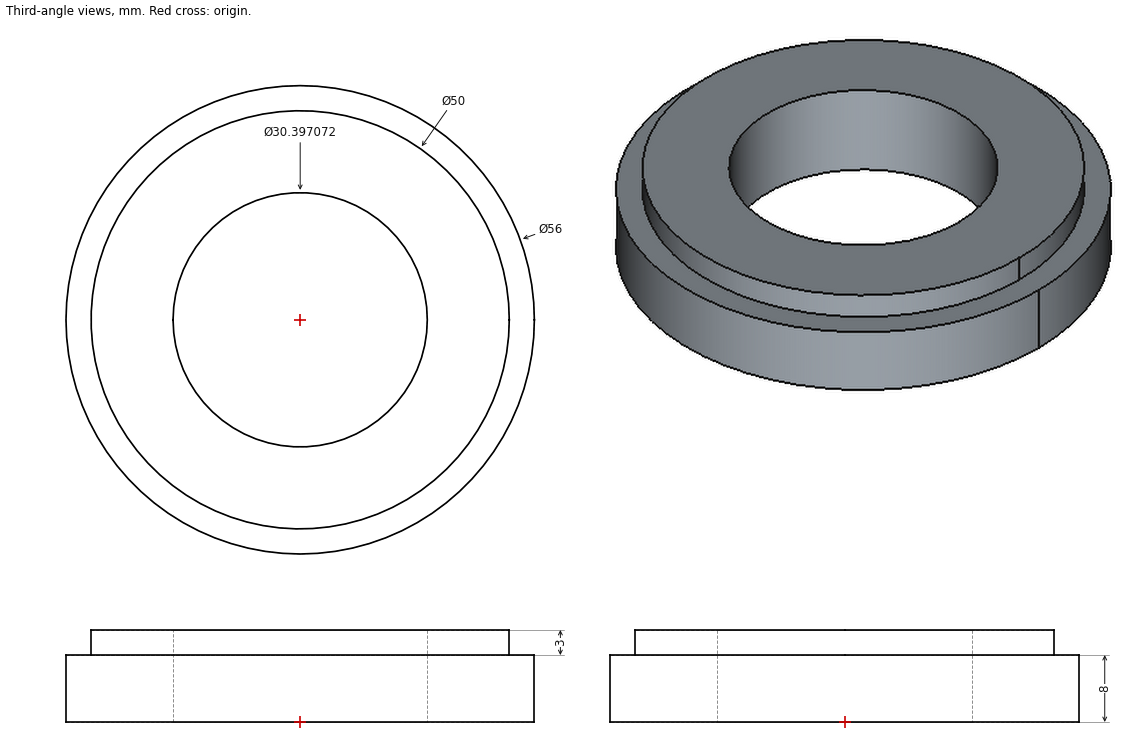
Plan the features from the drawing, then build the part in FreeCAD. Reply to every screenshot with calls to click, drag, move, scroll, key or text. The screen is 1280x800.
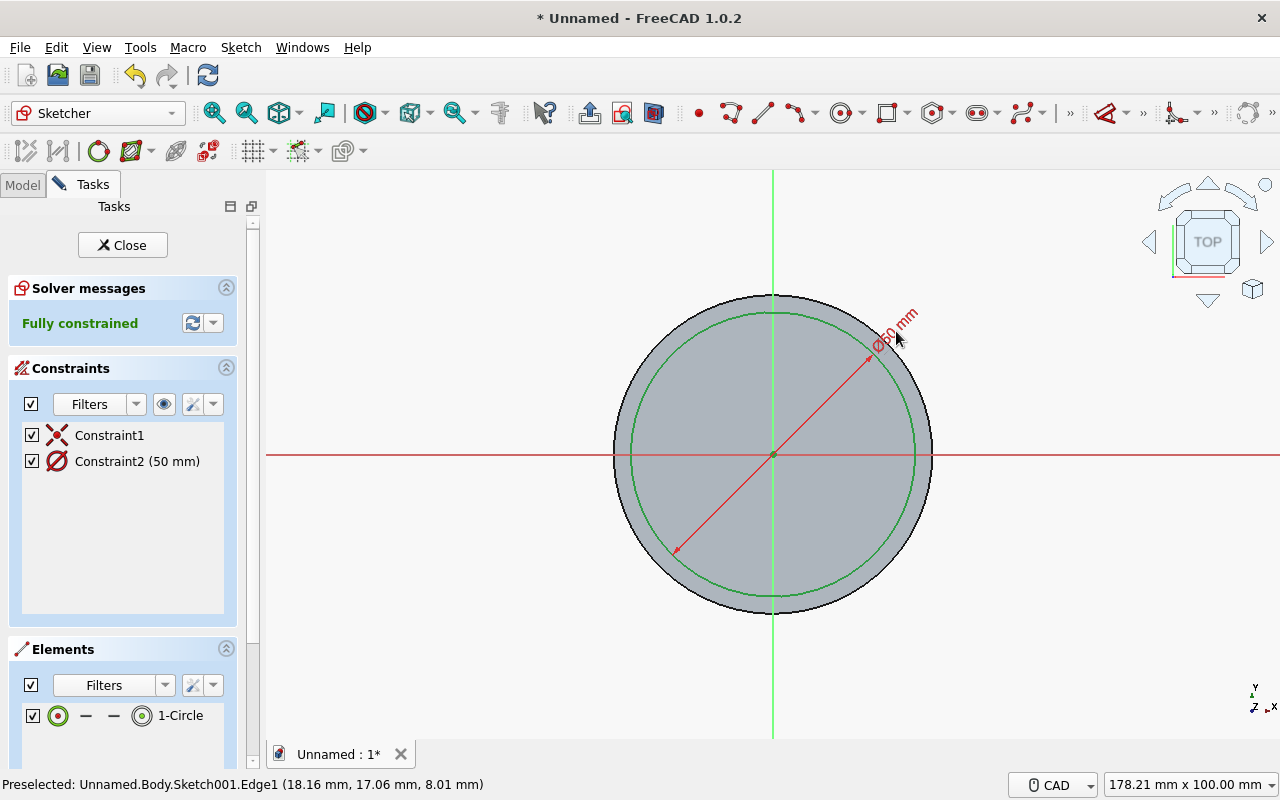
click(123, 245)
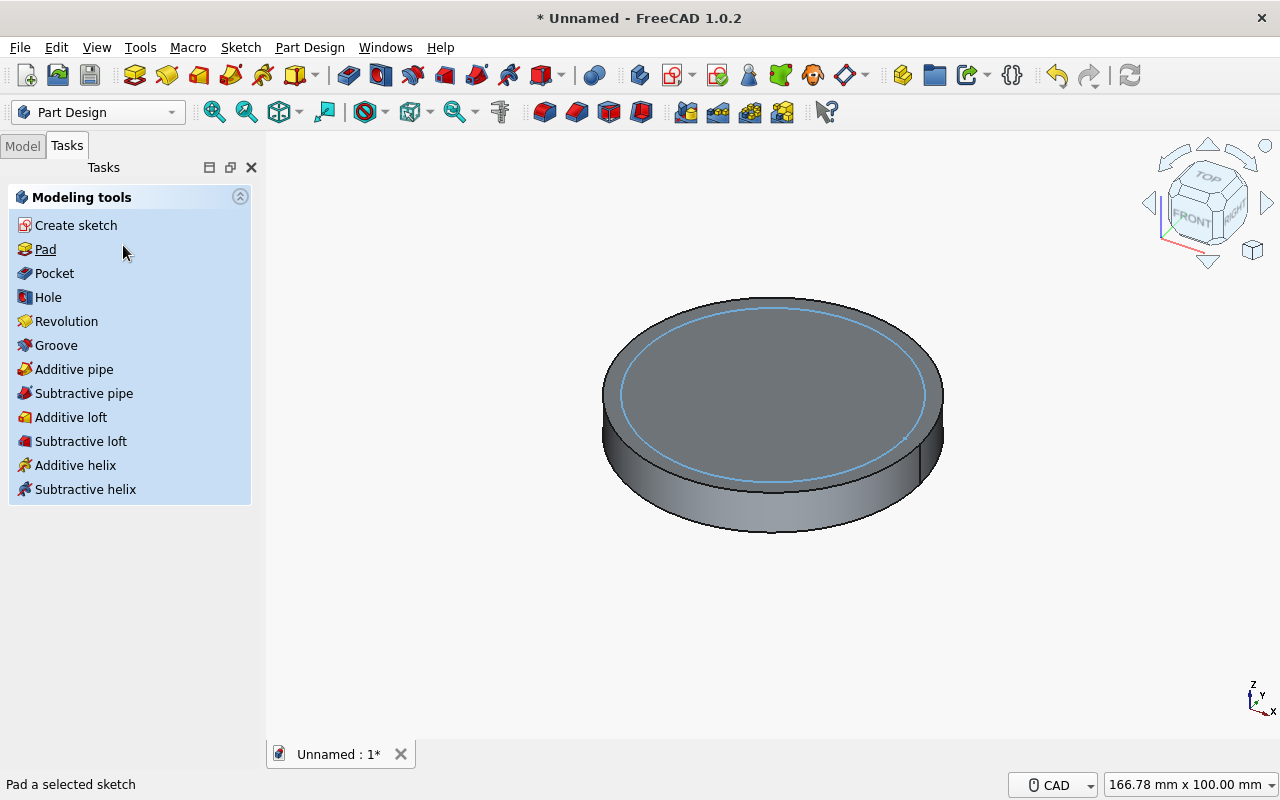
click(136, 76)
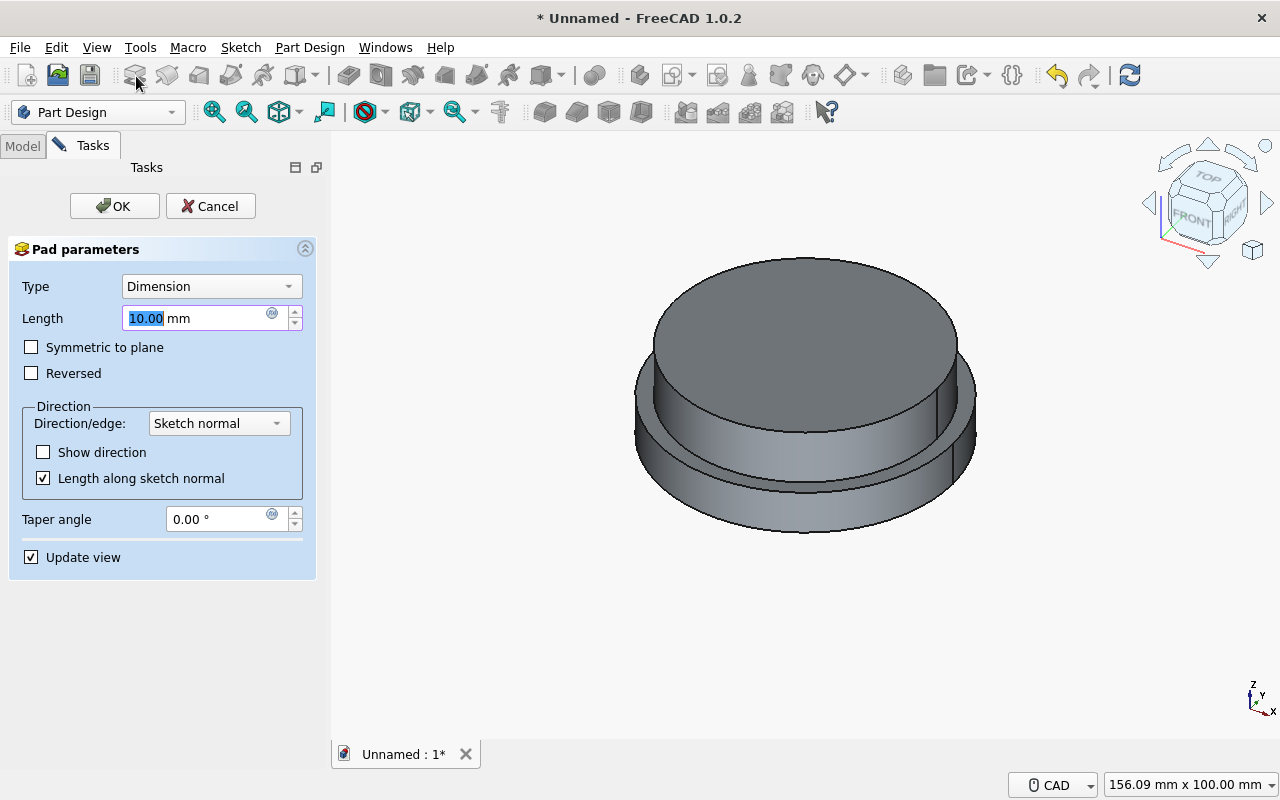
text(3)
key(Tab)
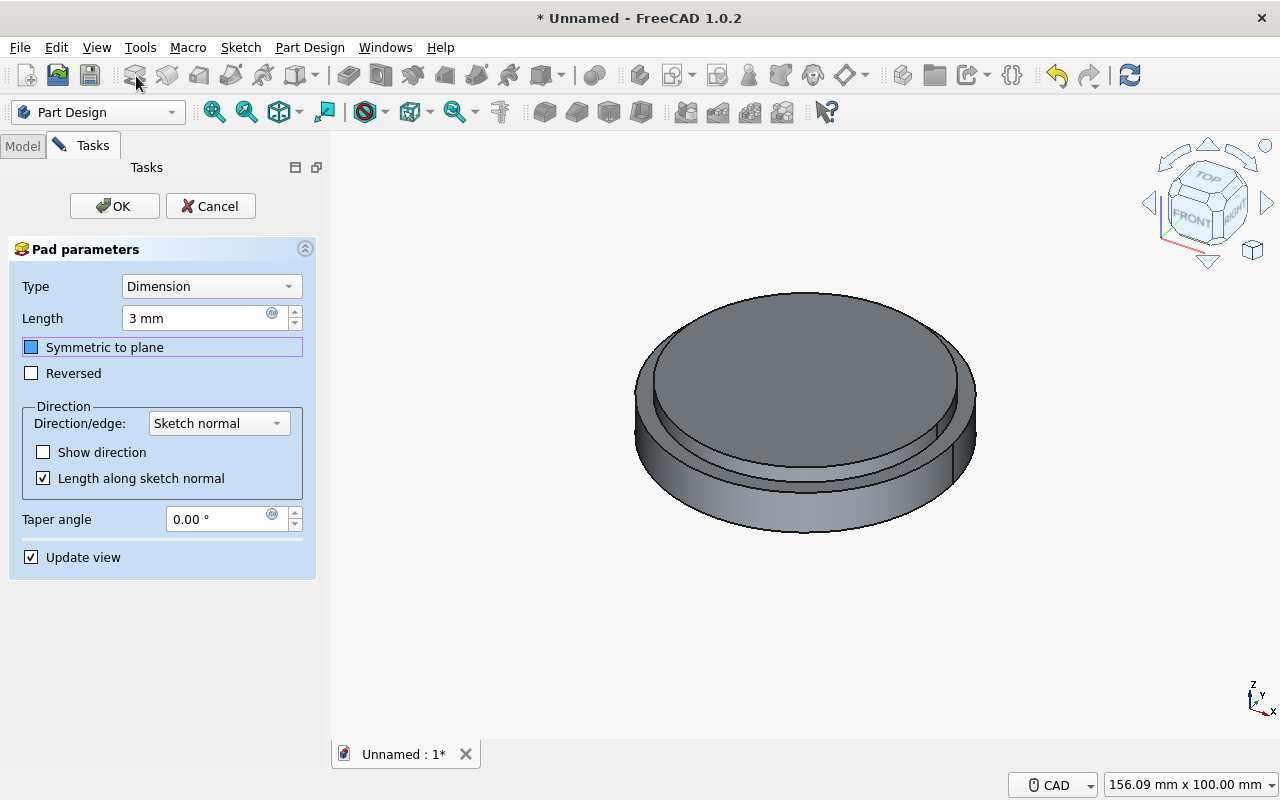
click(115, 206)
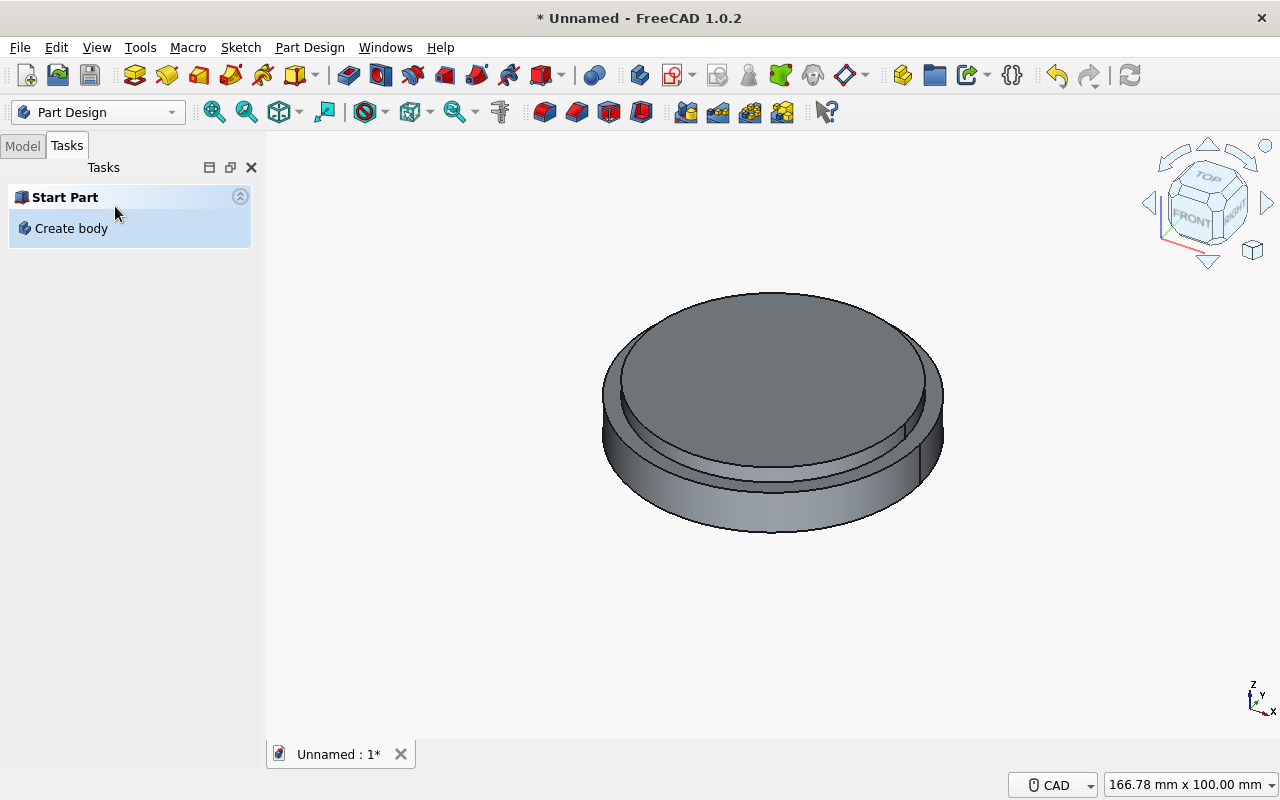
click(672, 76)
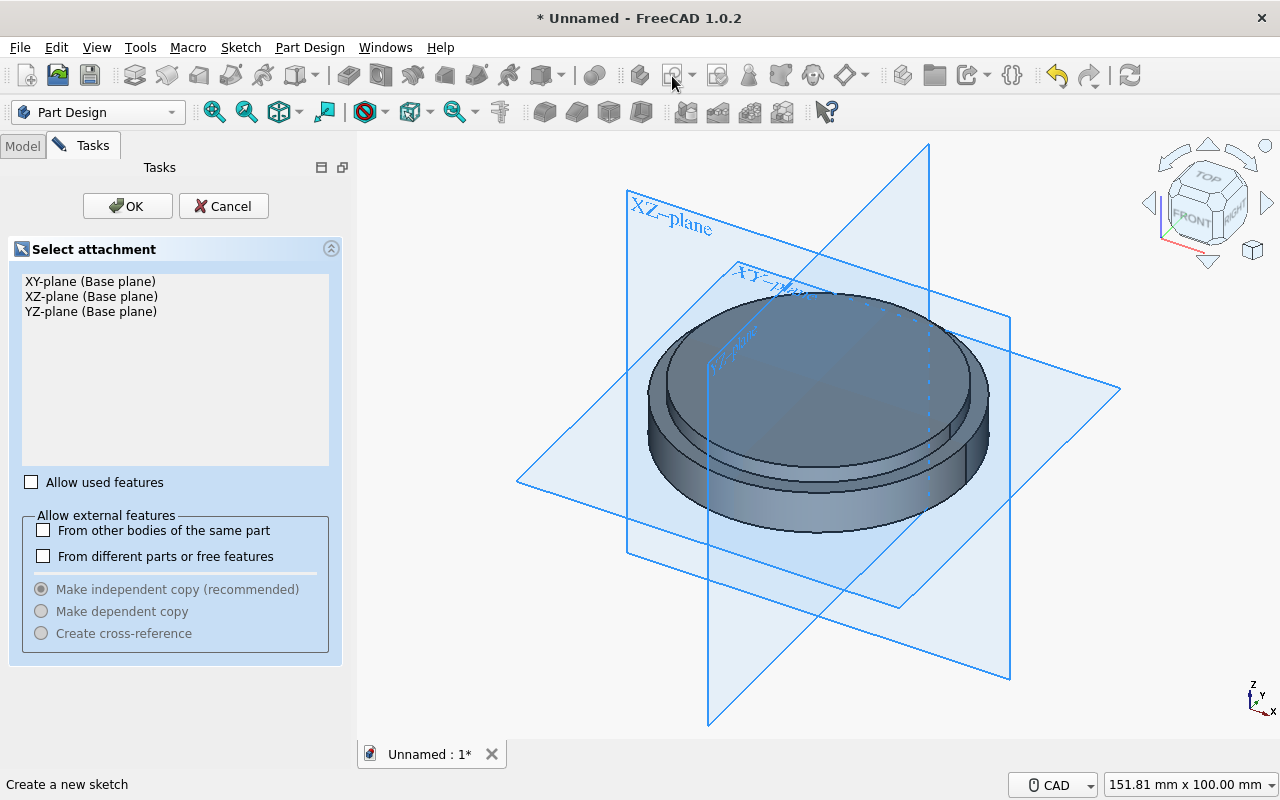
click(82, 282)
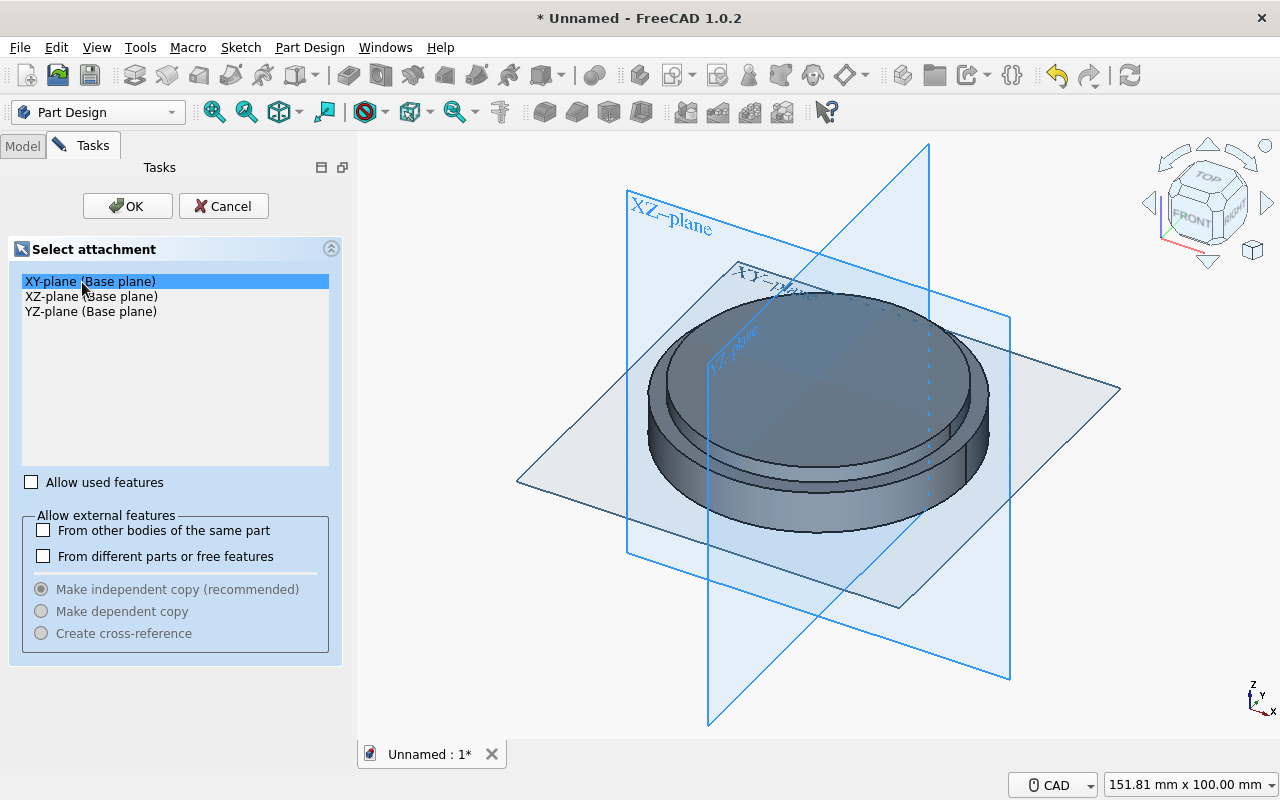
click(128, 206)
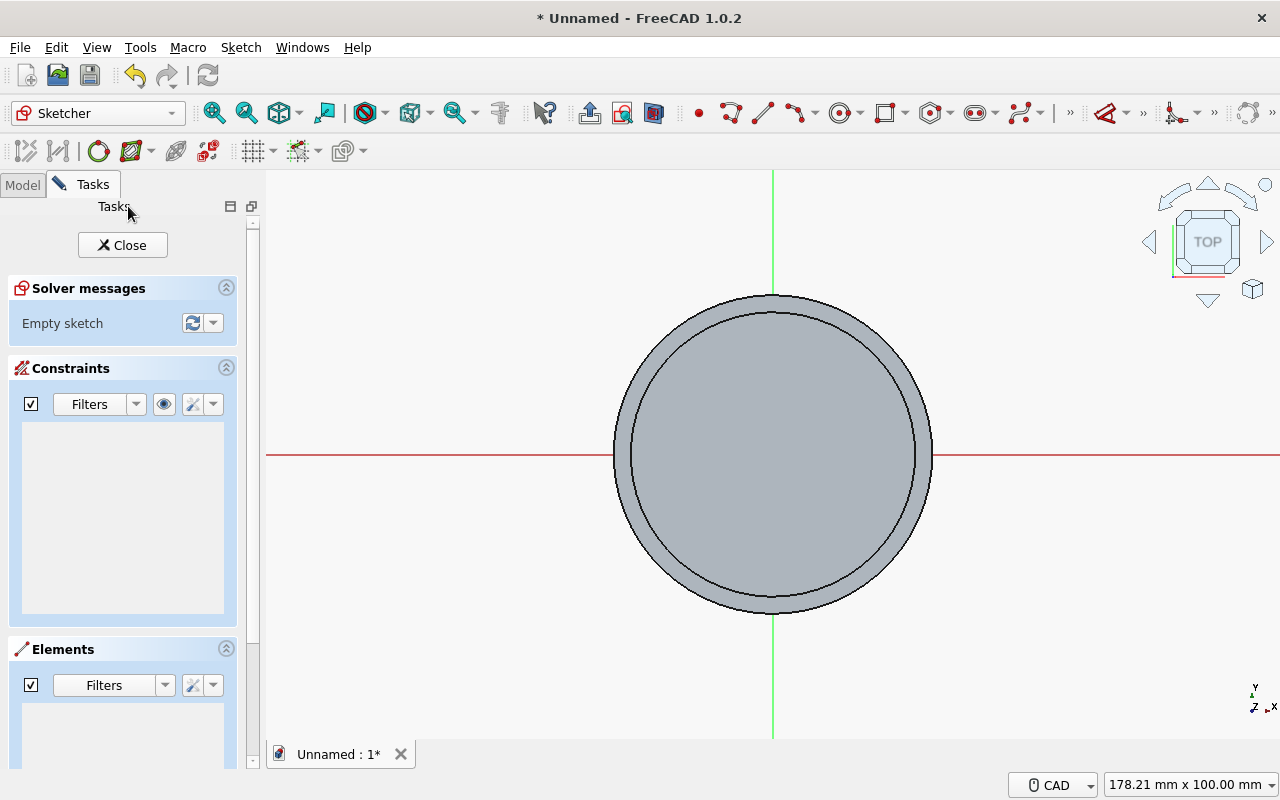
click(654, 114)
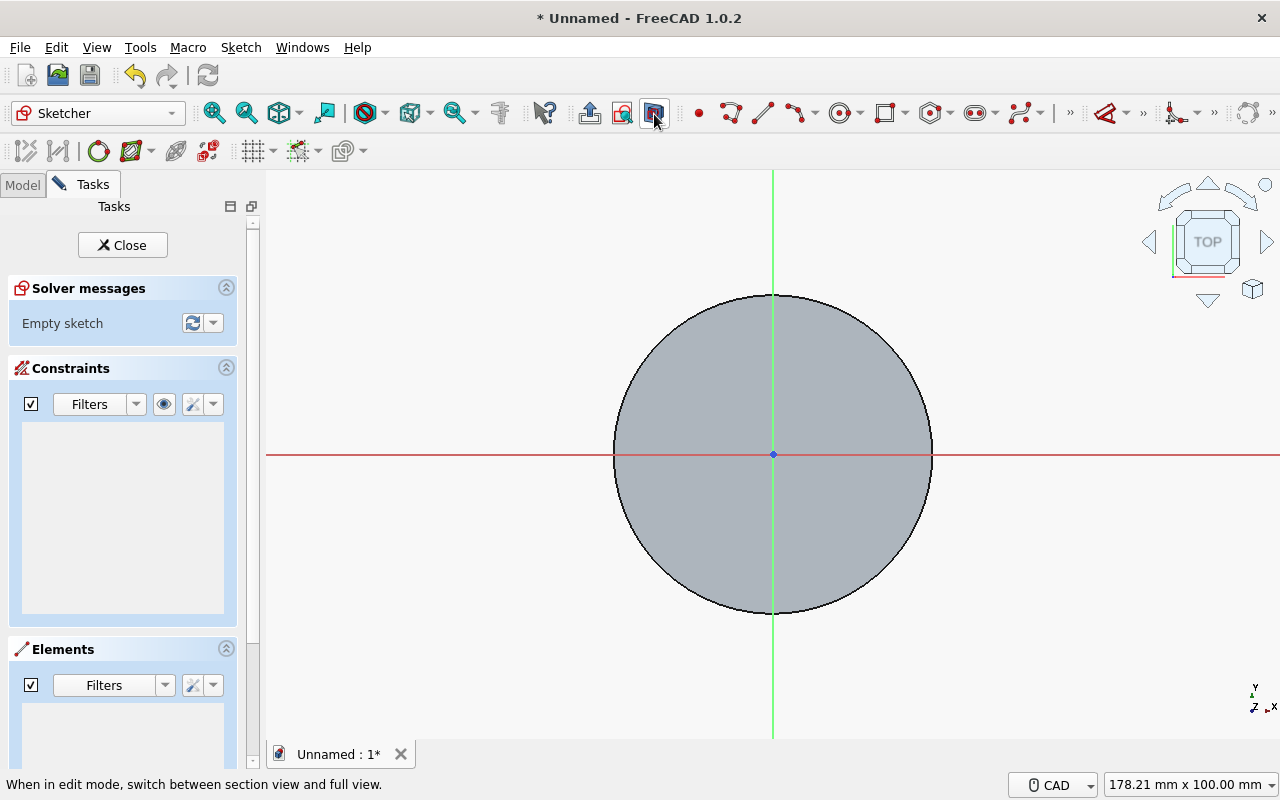
scroll(829, 455, up, 4)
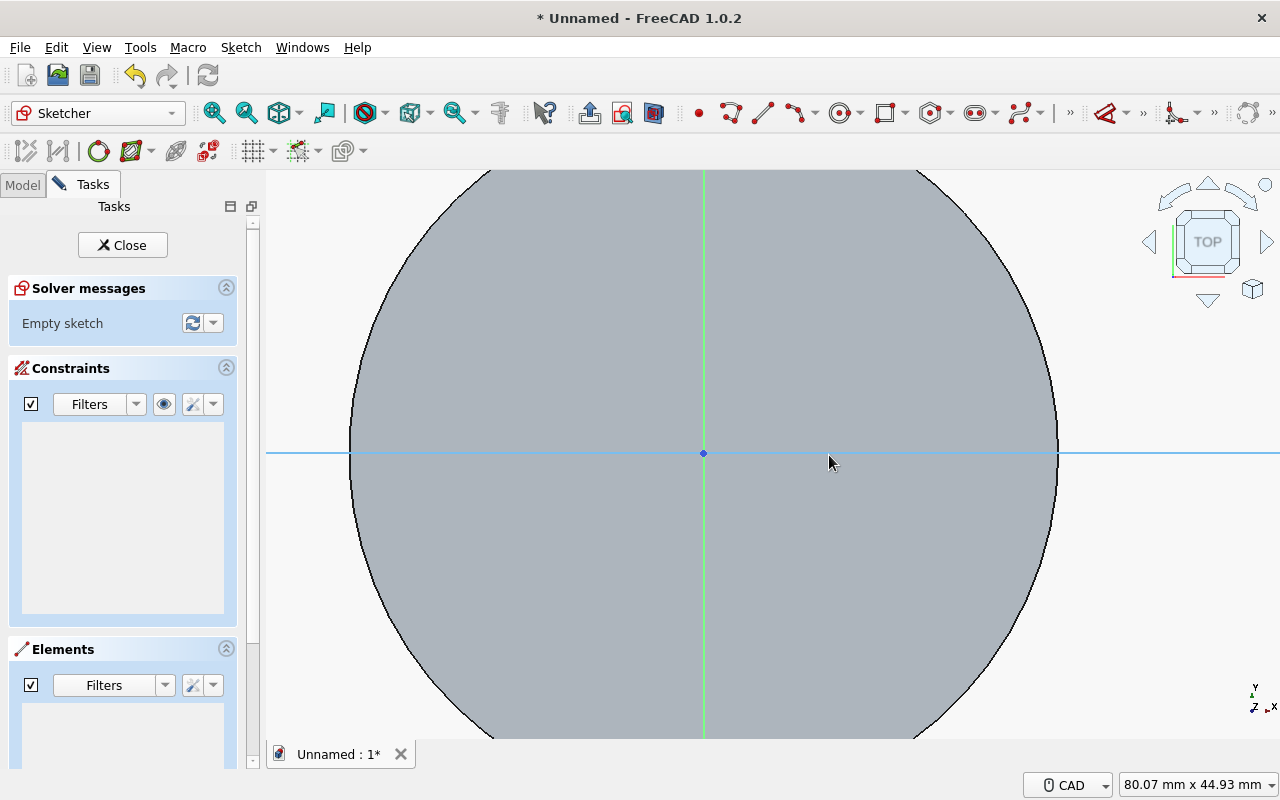
click(840, 114)